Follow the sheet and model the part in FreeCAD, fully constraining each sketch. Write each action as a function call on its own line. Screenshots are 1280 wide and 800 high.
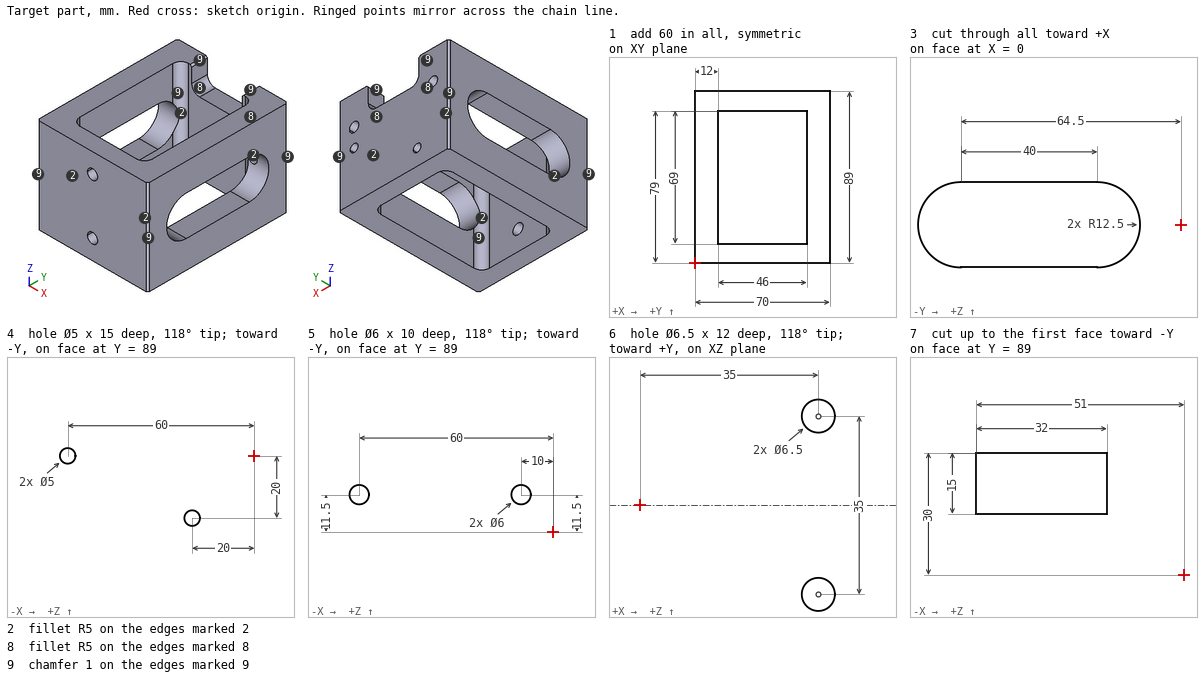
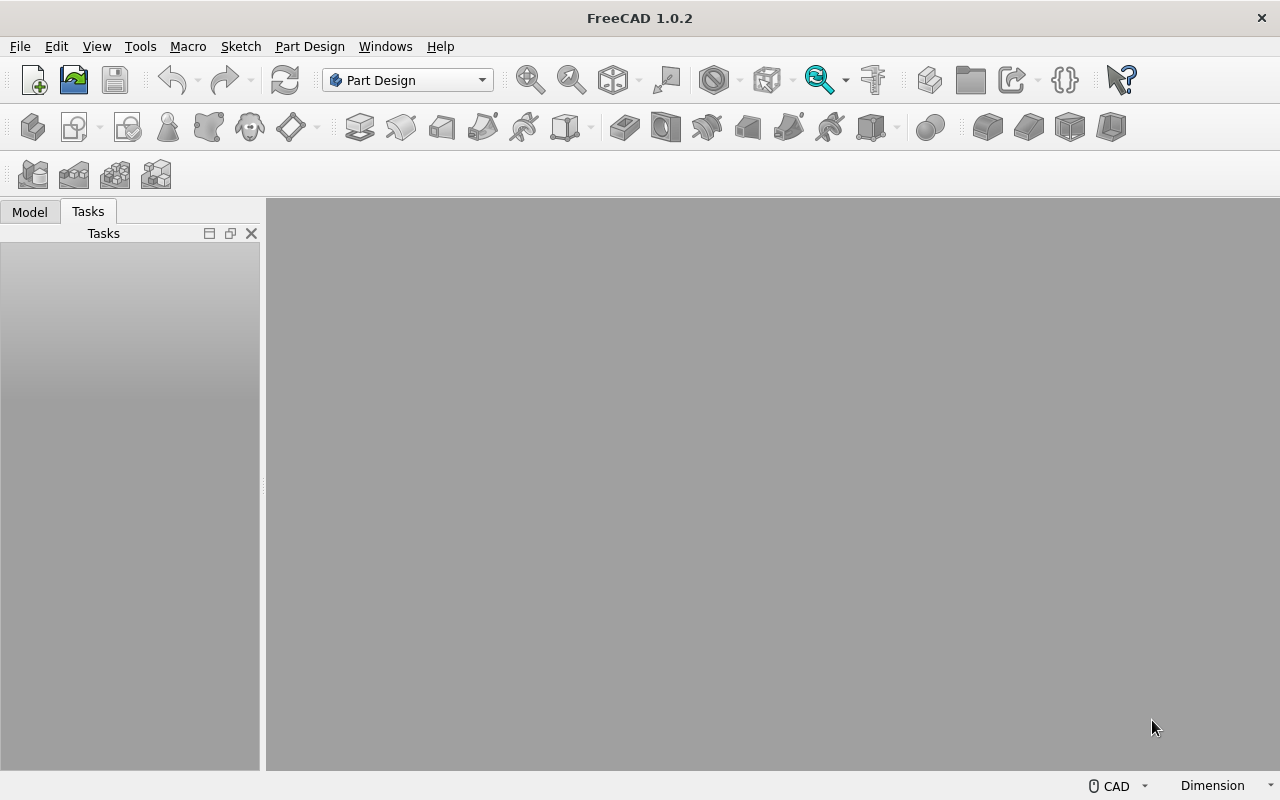
click(33, 80)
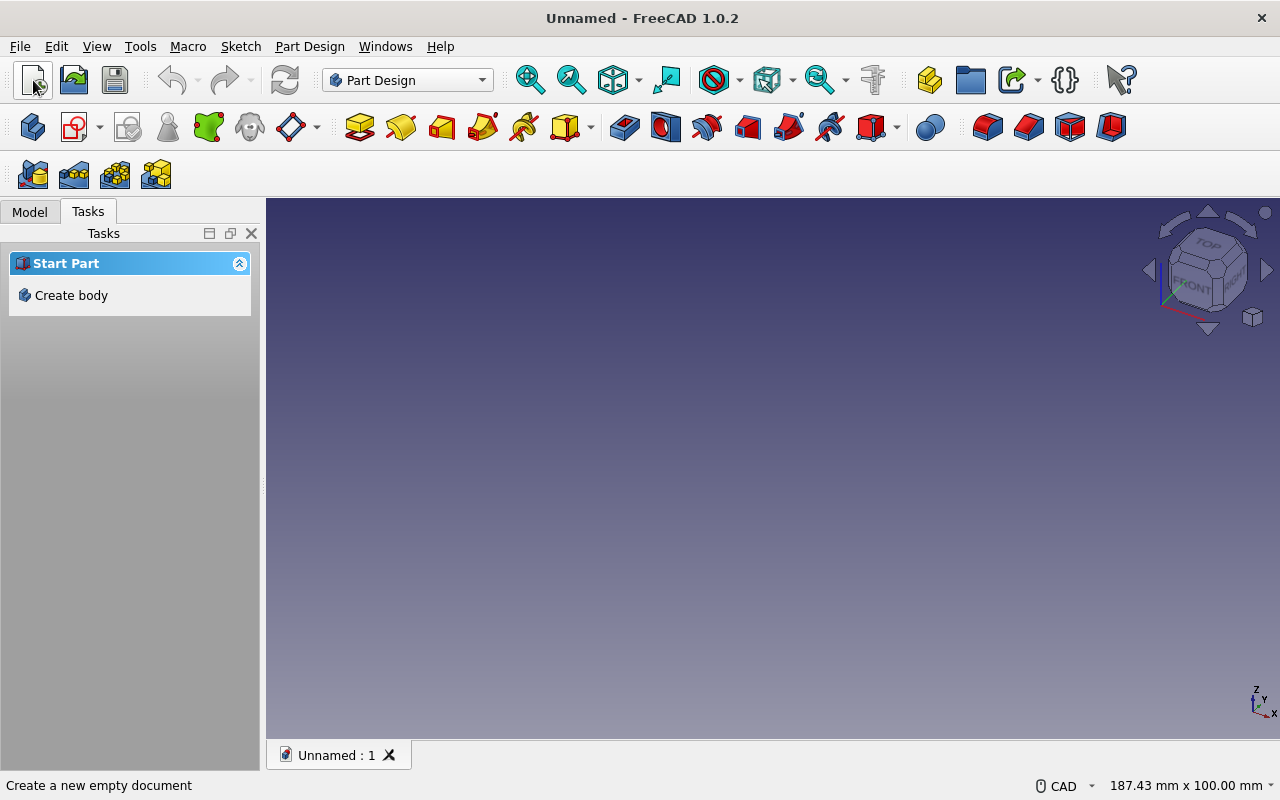
click(74, 128)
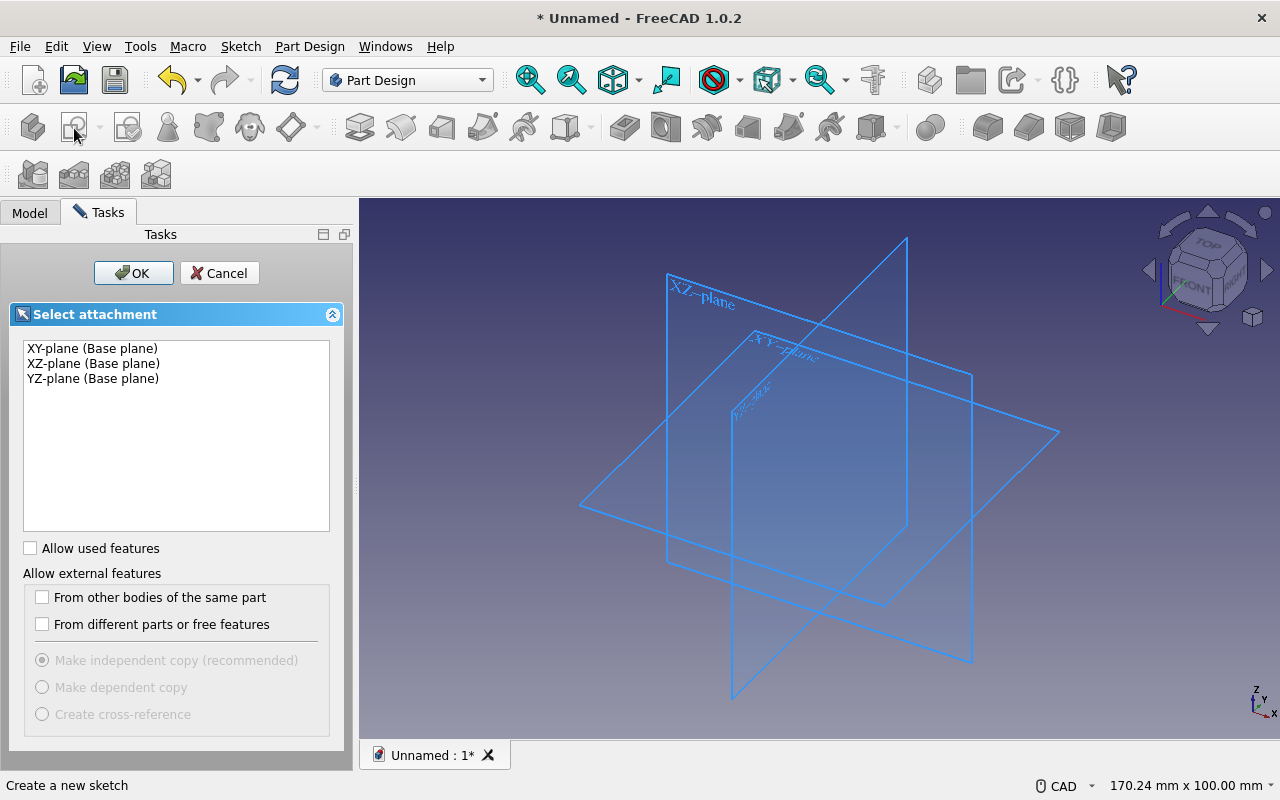
click(84, 348)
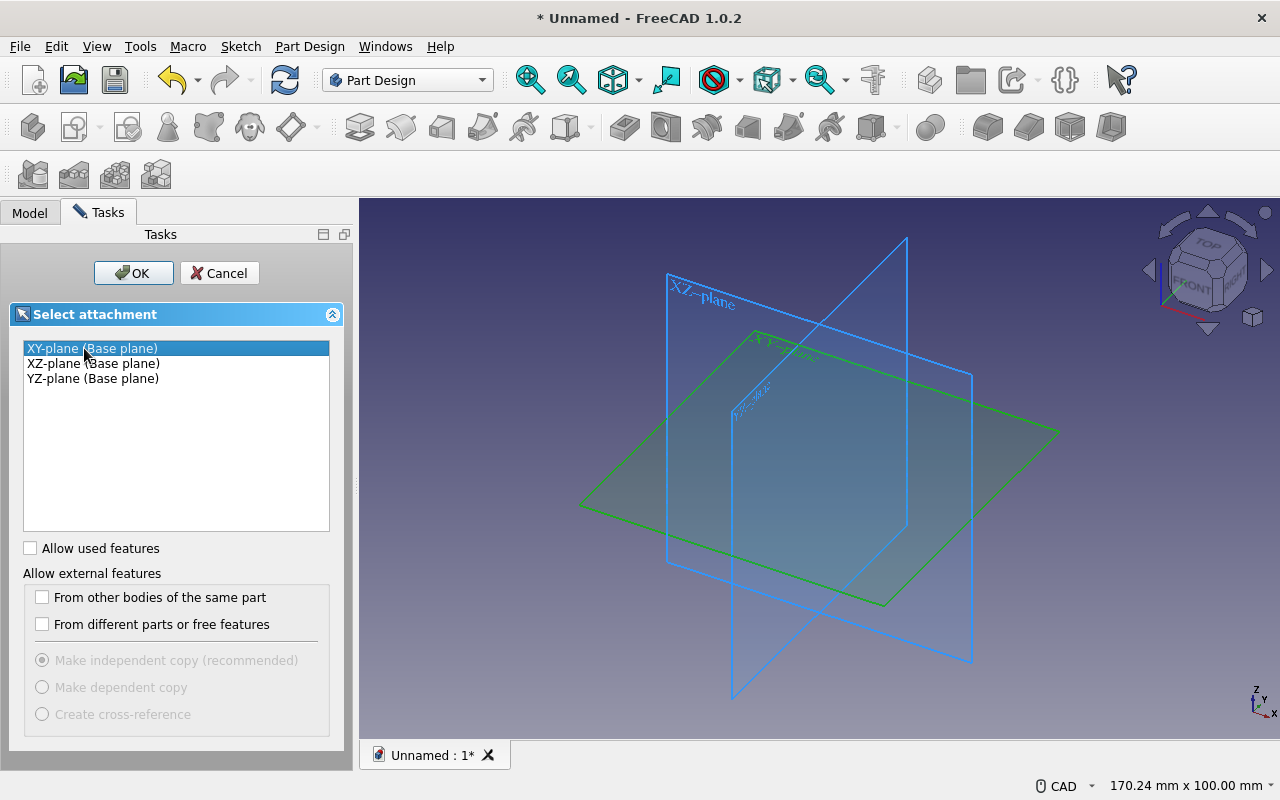
click(134, 273)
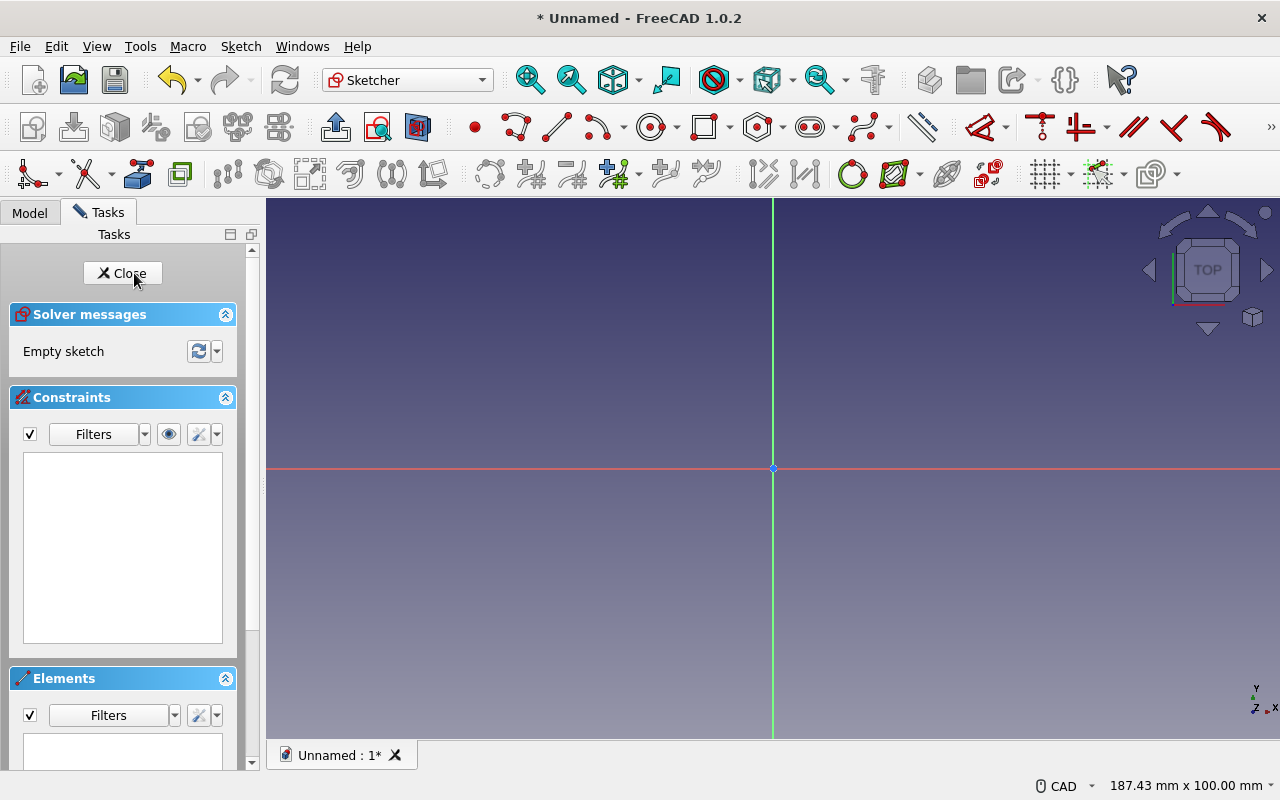
scroll(391, 711, down, 3)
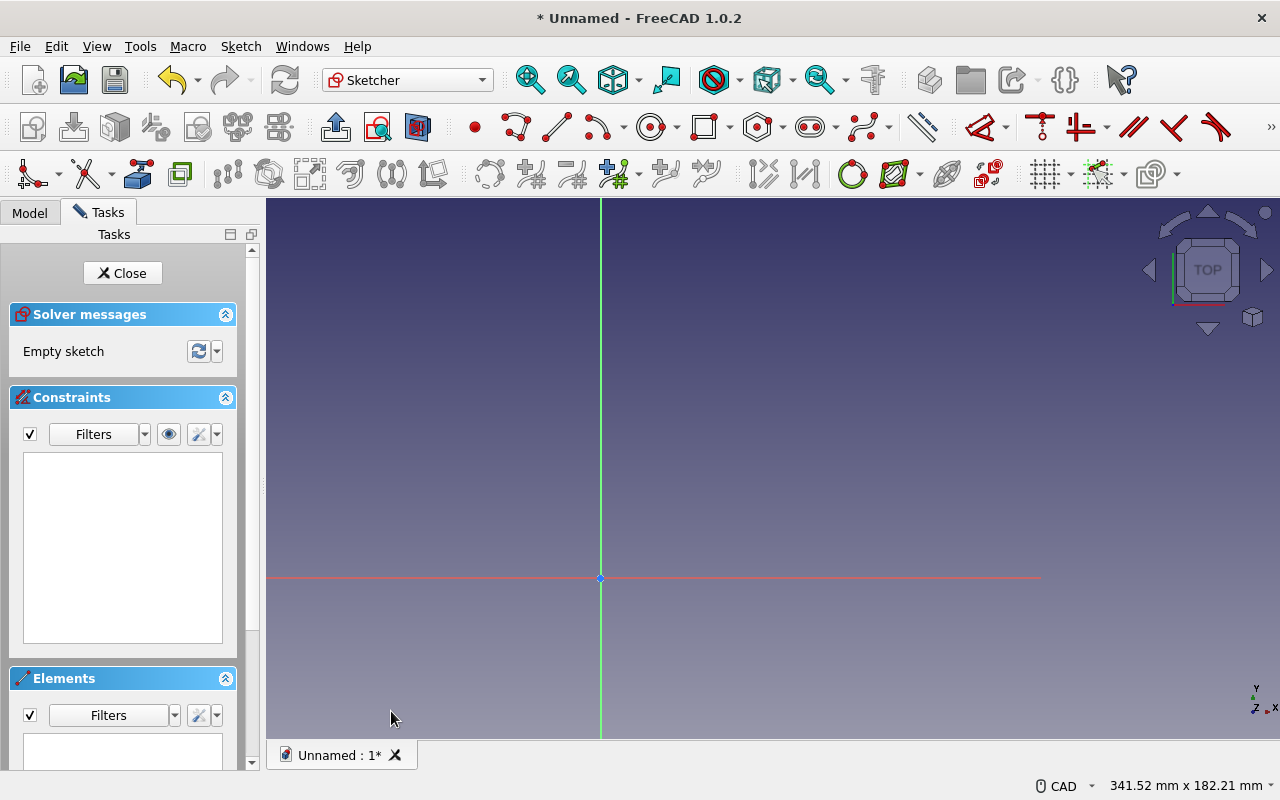
click(704, 128)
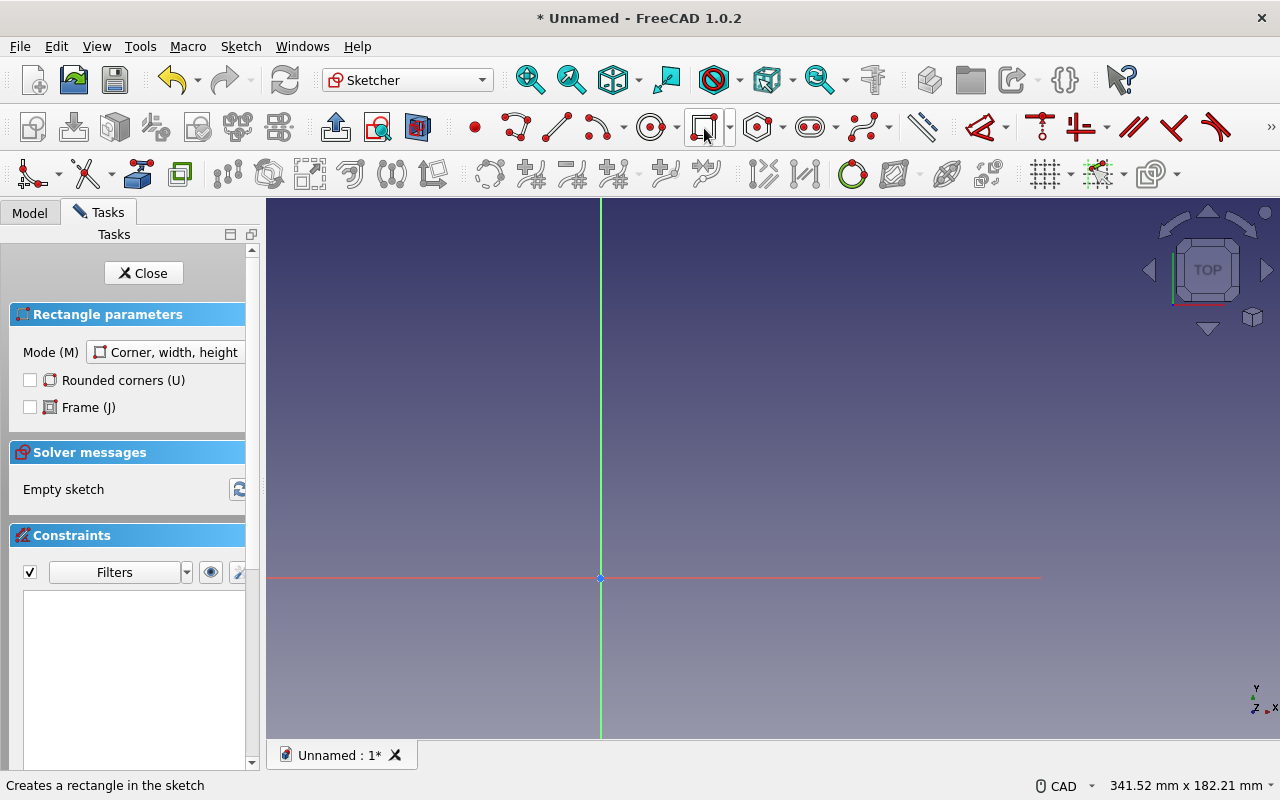
click(601, 578)
click(809, 314)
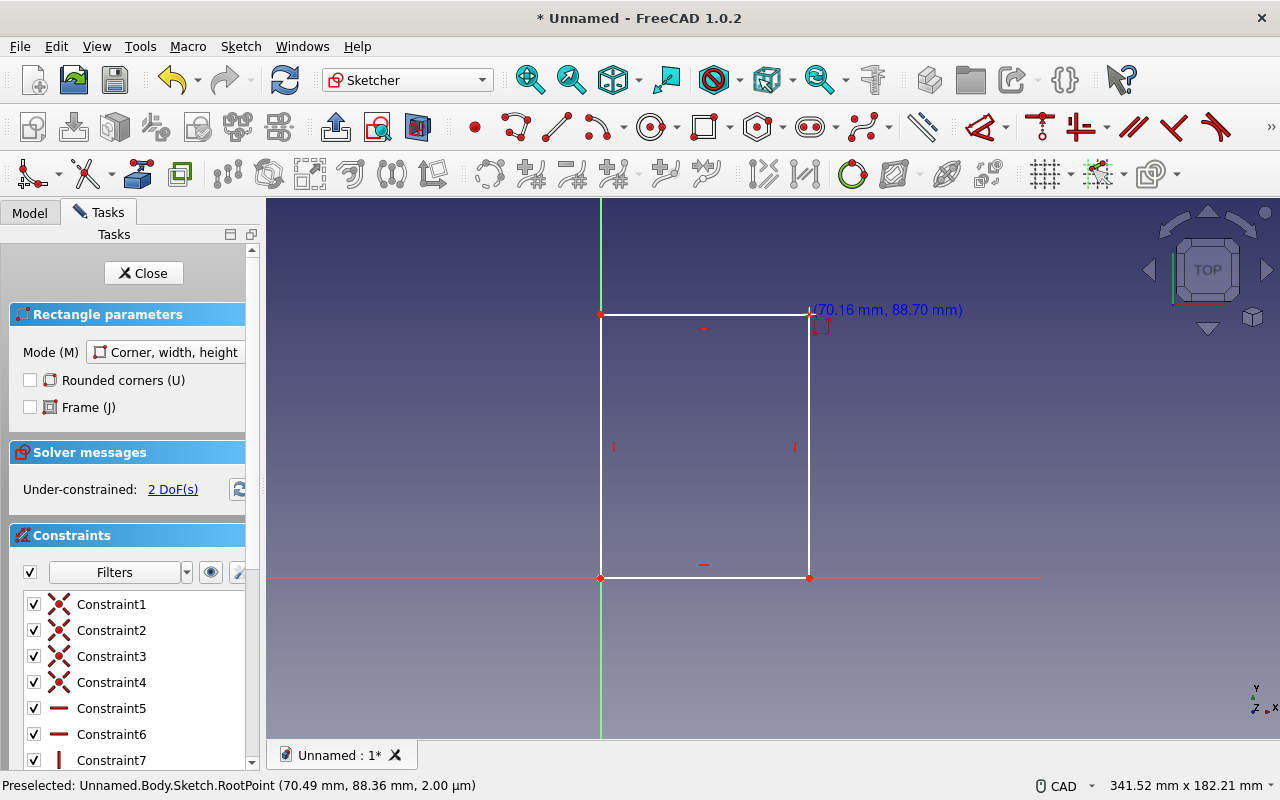
click(636, 344)
click(773, 549)
key(Escape)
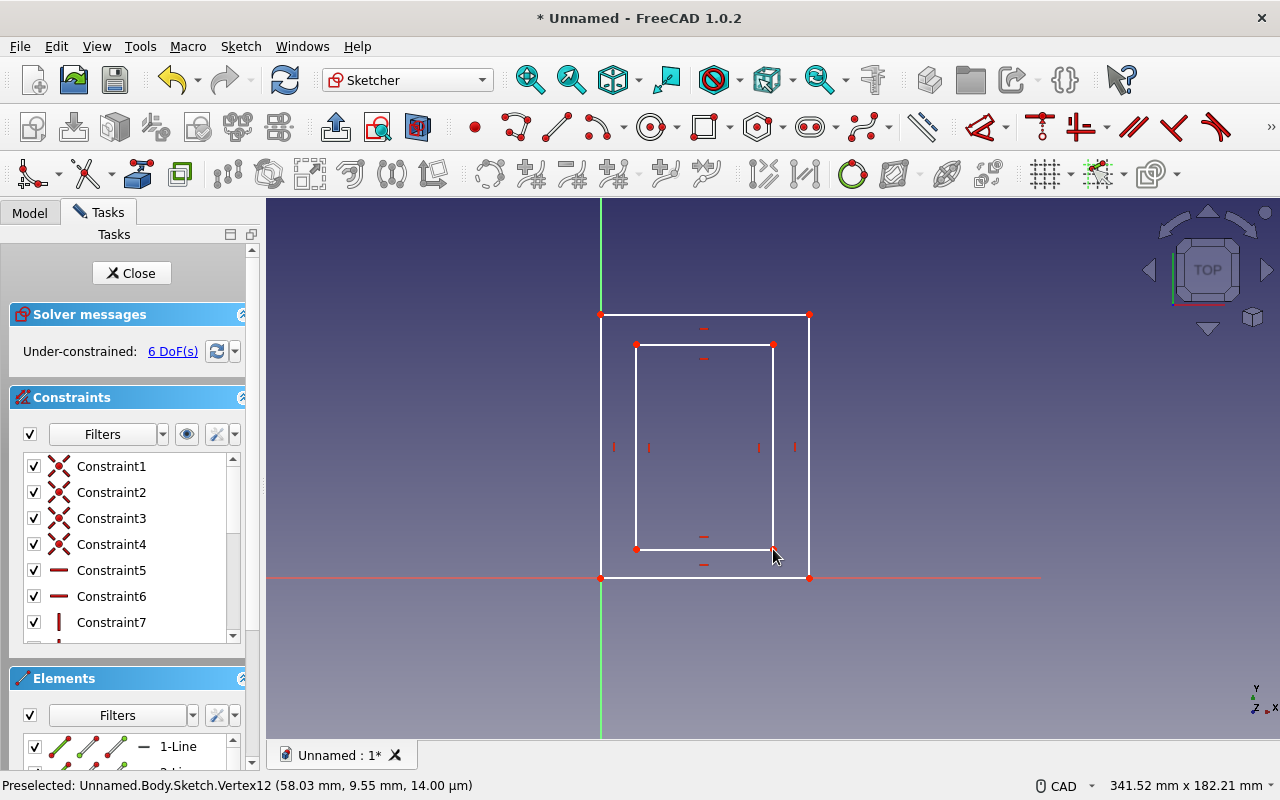
key(d)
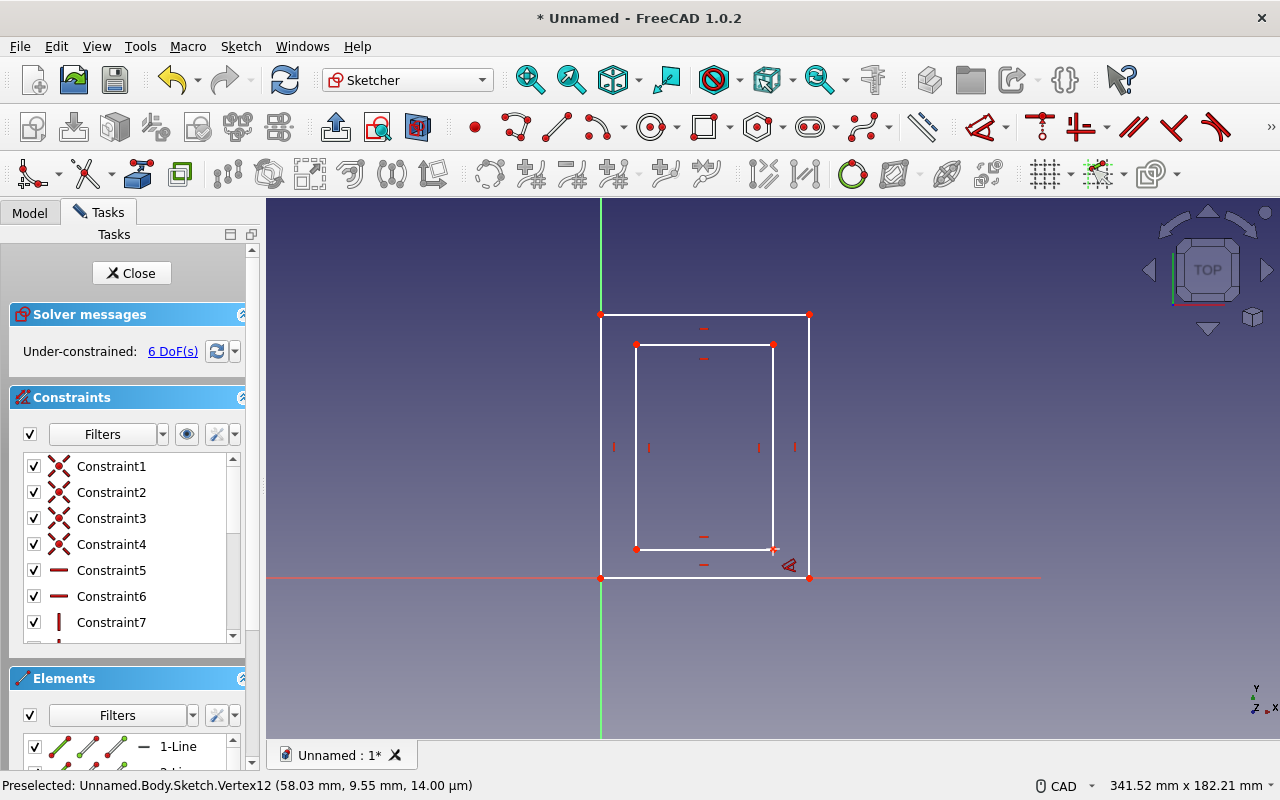
click(663, 578)
click(705, 612)